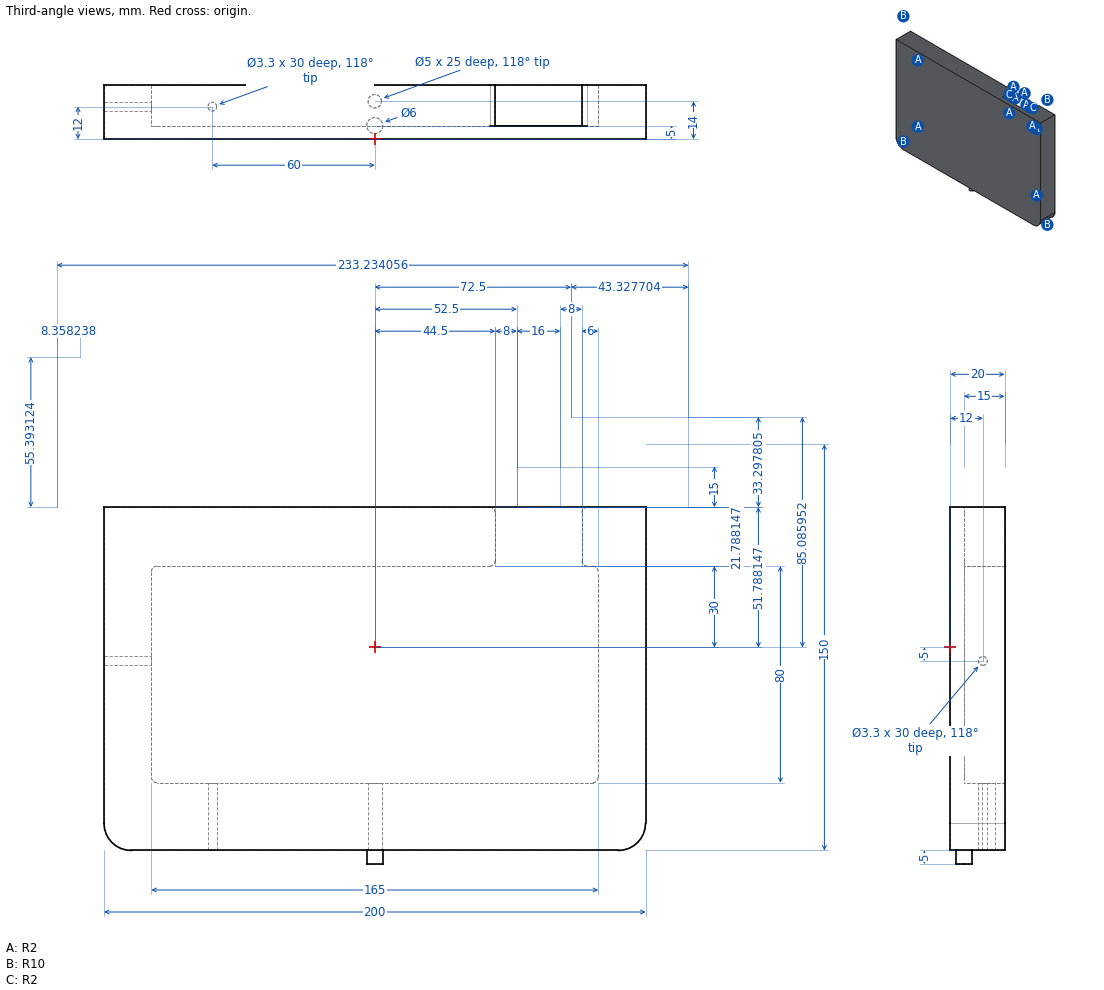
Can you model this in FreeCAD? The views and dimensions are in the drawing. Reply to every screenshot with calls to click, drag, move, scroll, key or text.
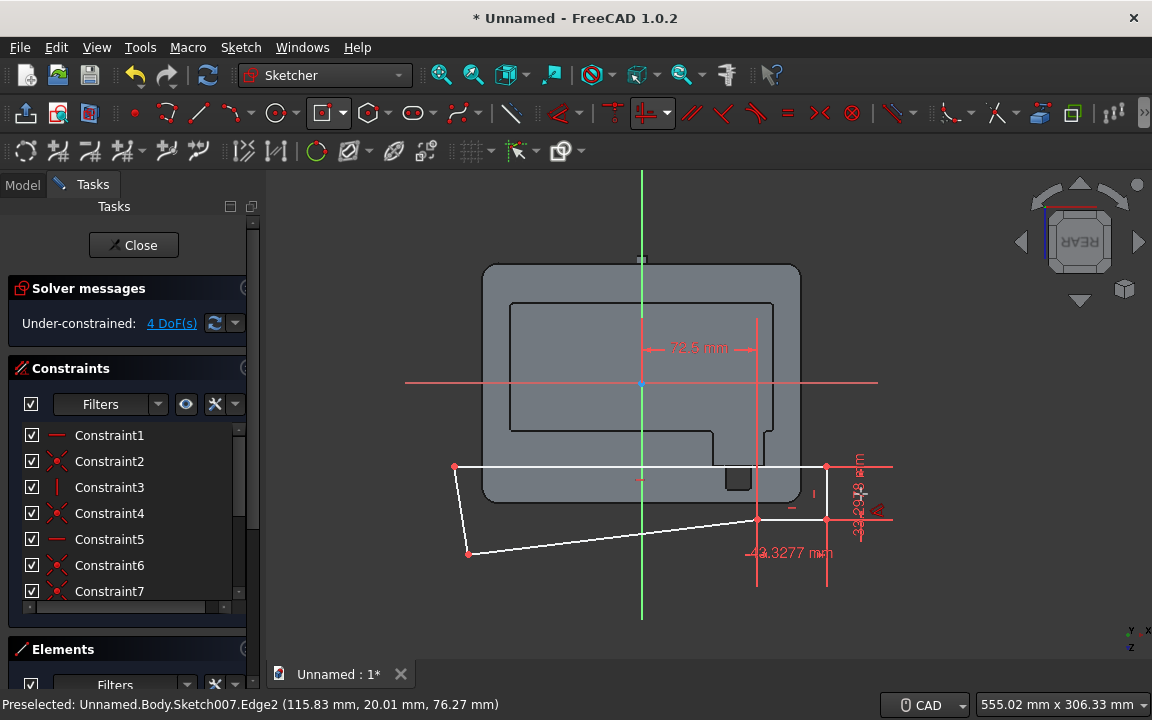
scroll(458, 493, up, 6)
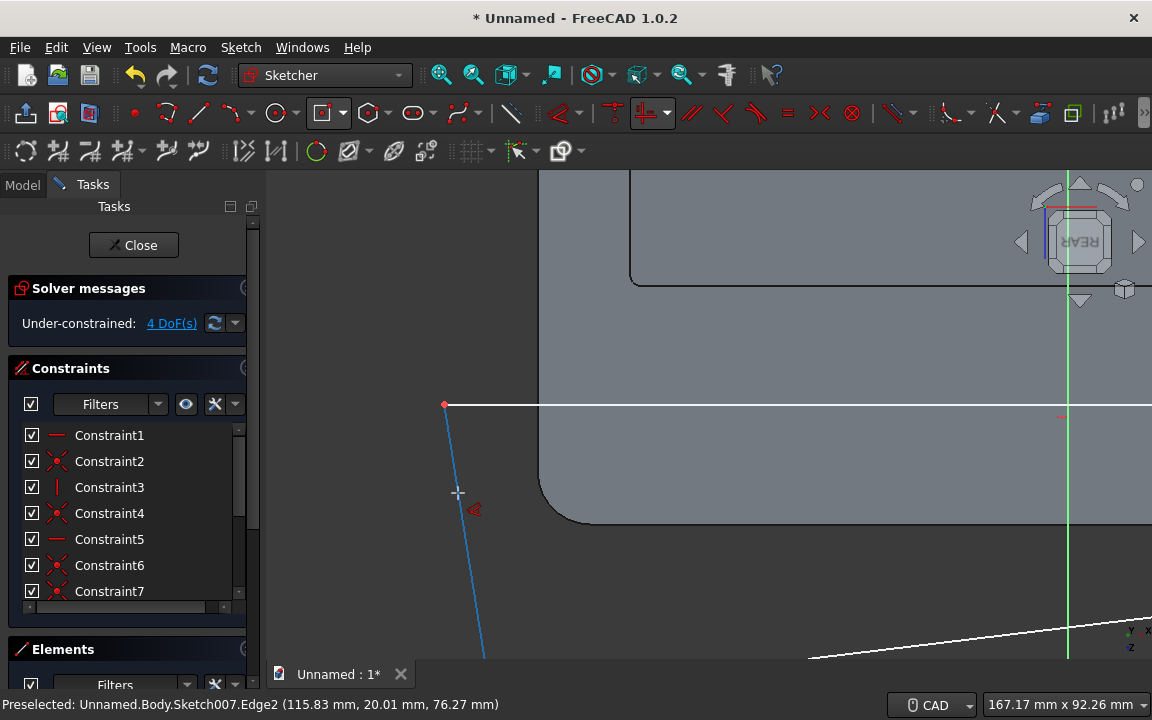
click(458, 492)
click(467, 371)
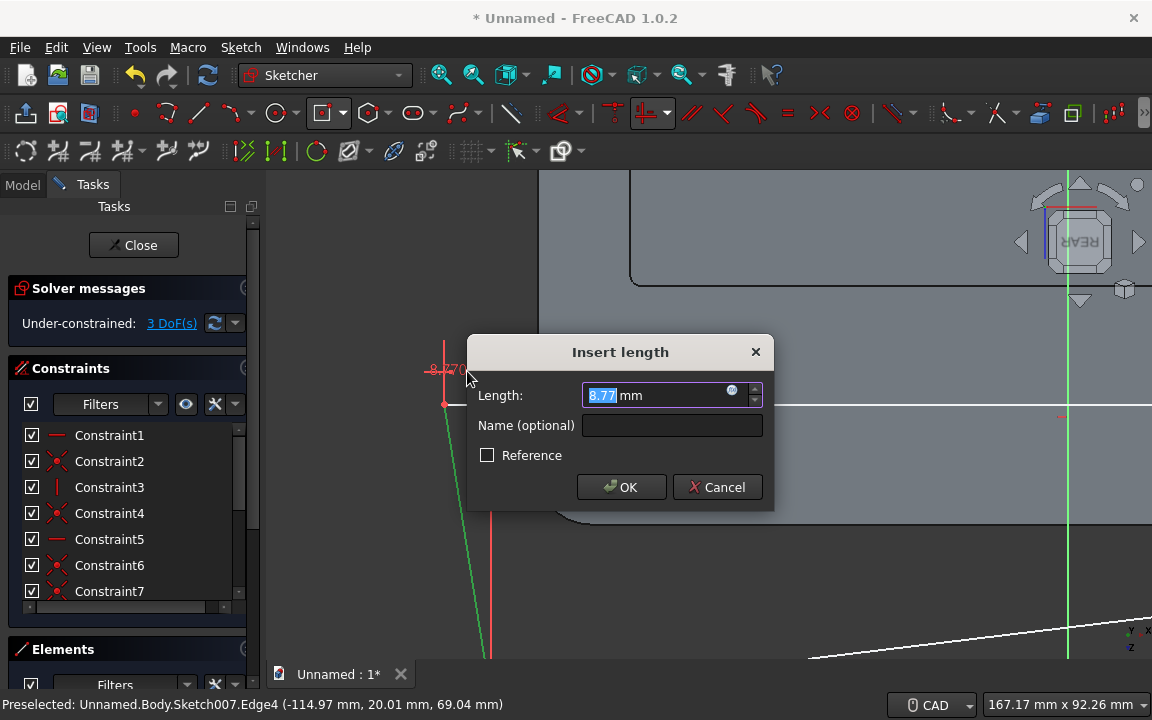
text(8.358238)
key(Return)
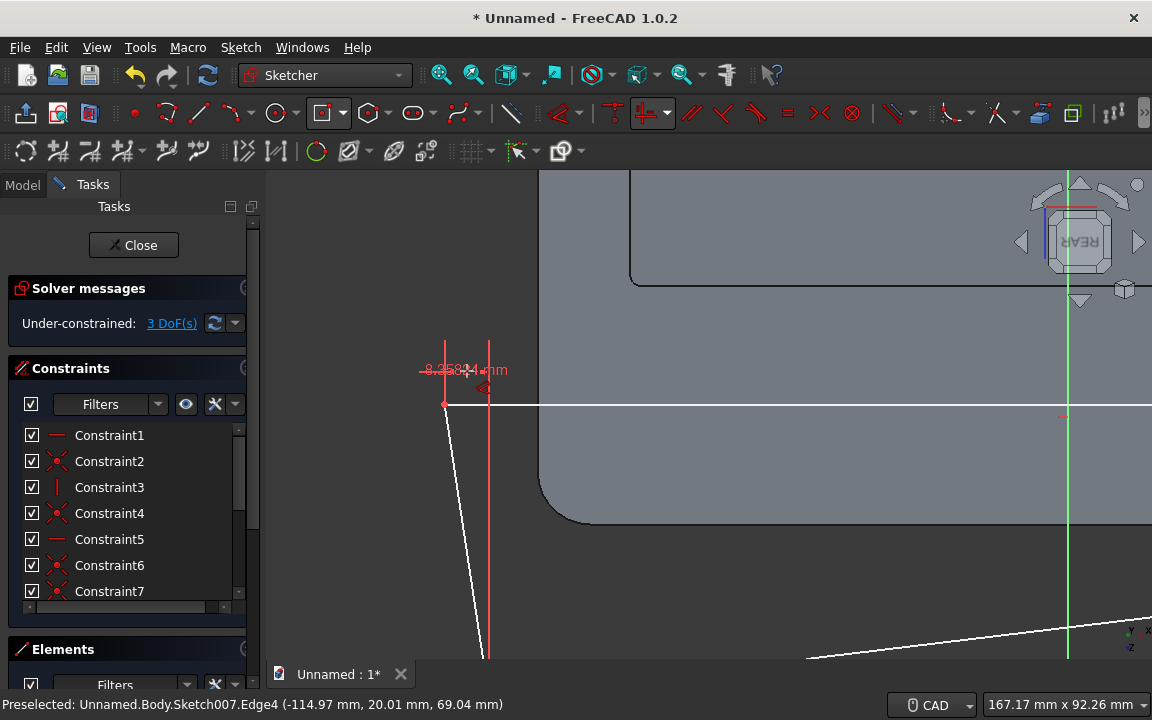
click(816, 405)
click(716, 371)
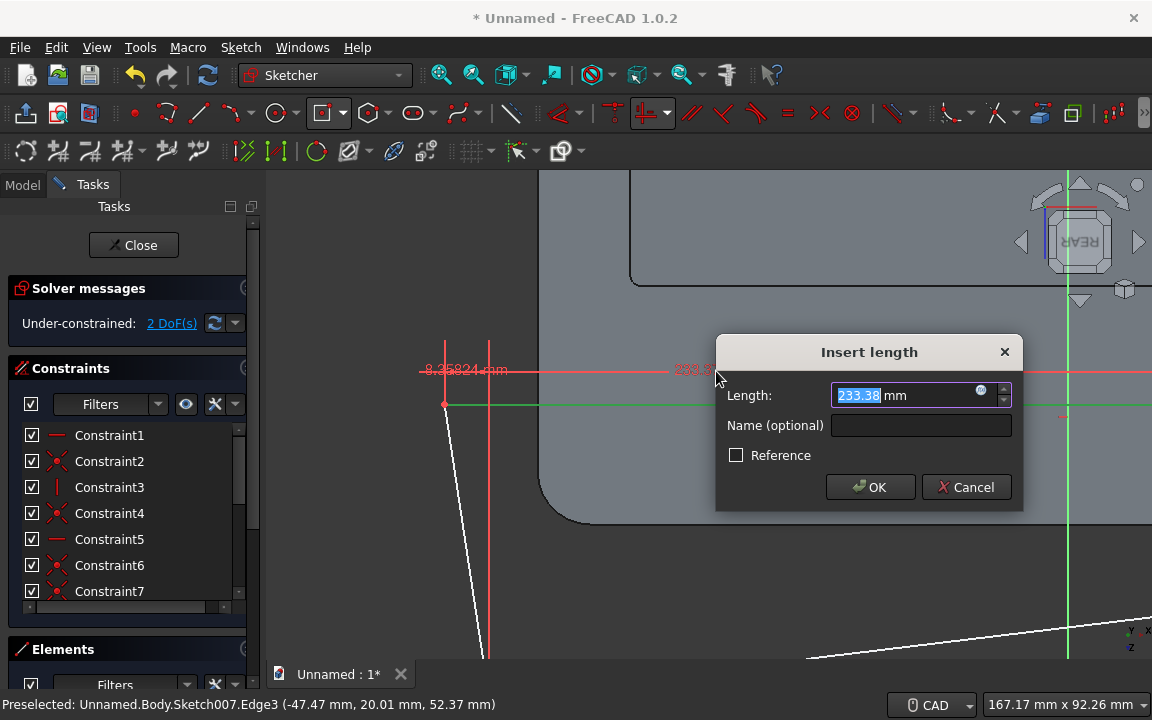
text(233.234056)
key(Return)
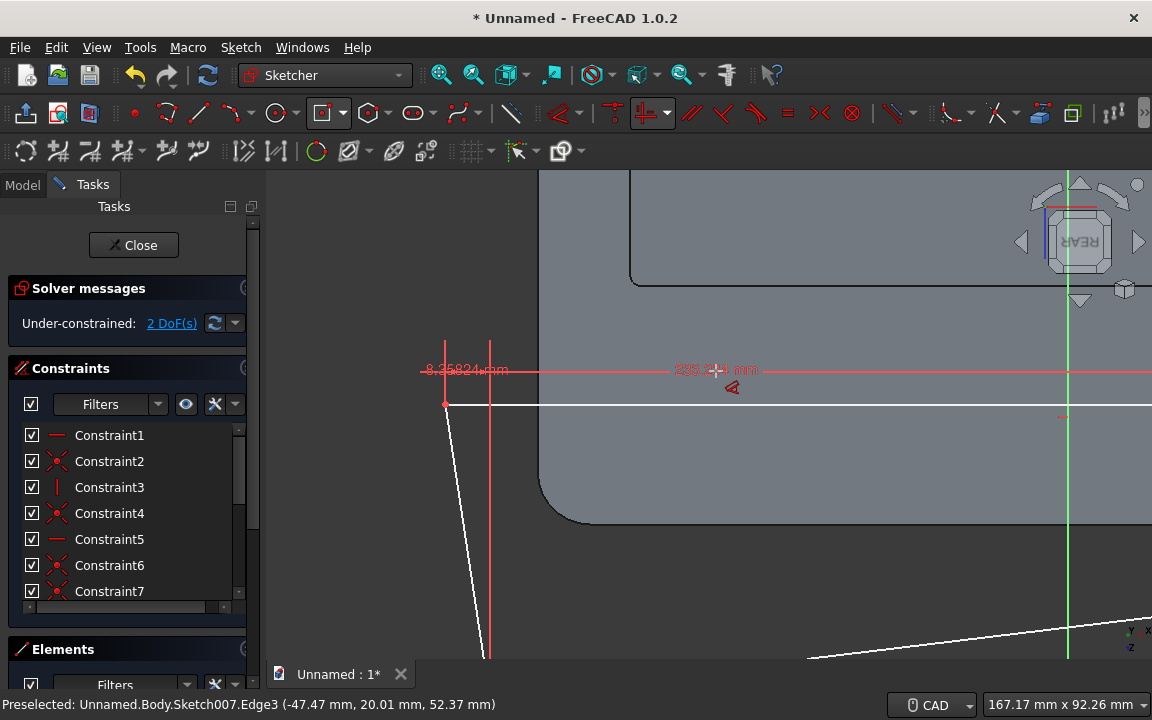
scroll(394, 416, down, 5)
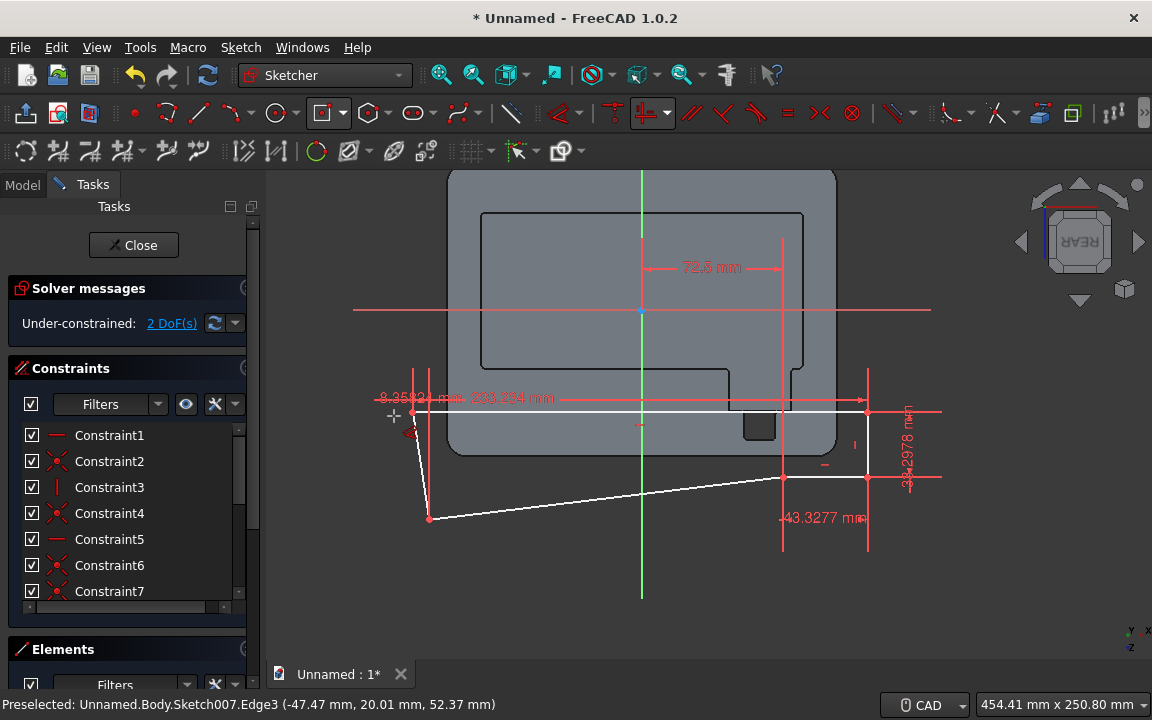
click(783, 477)
click(817, 394)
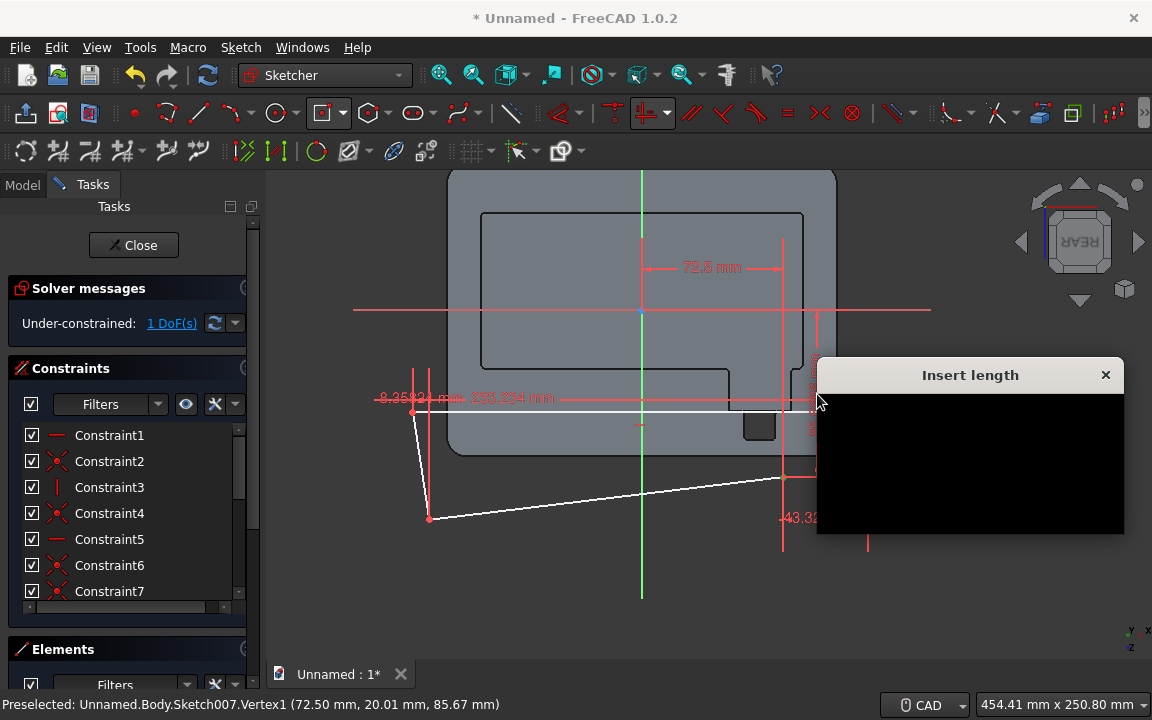
text(85.085952)
key(Return)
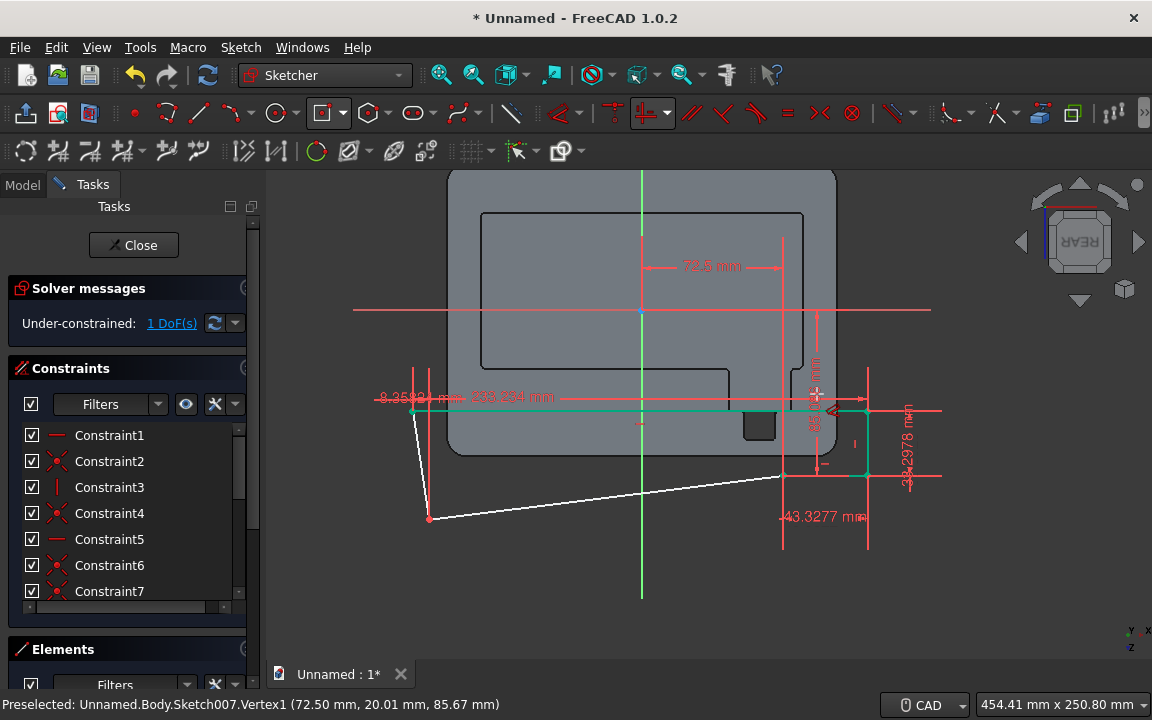
click(418, 444)
click(379, 465)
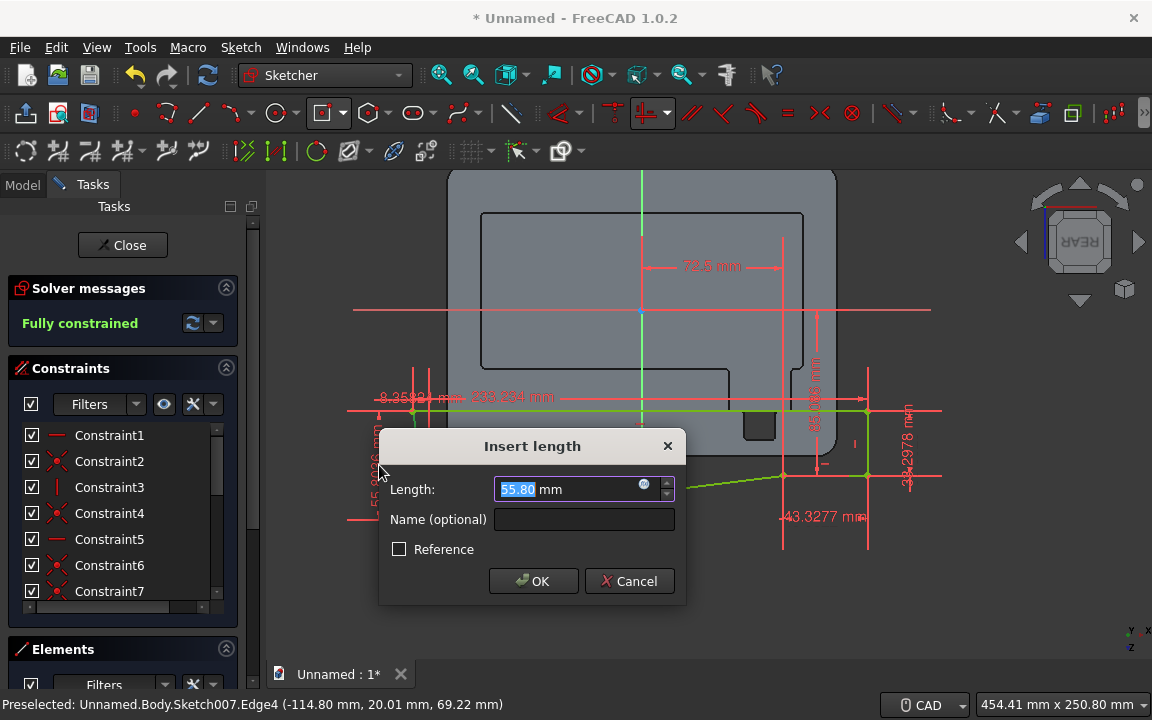
text(55.393124)
key(Return)
key(Escape)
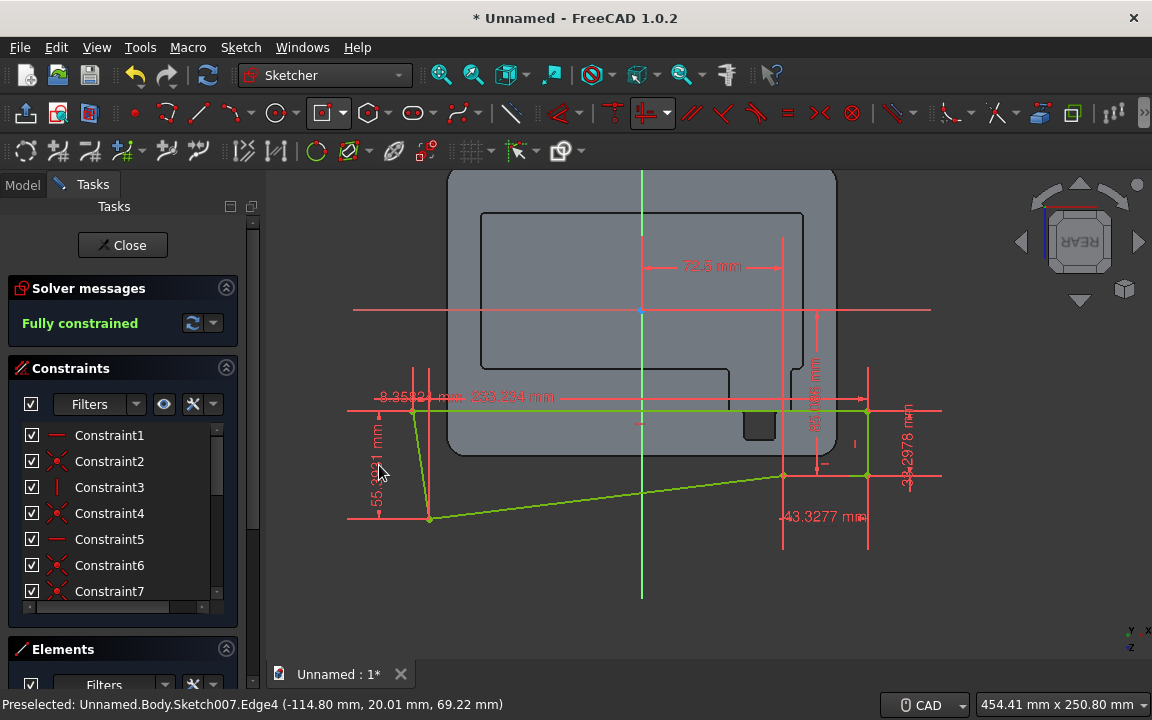
click(123, 245)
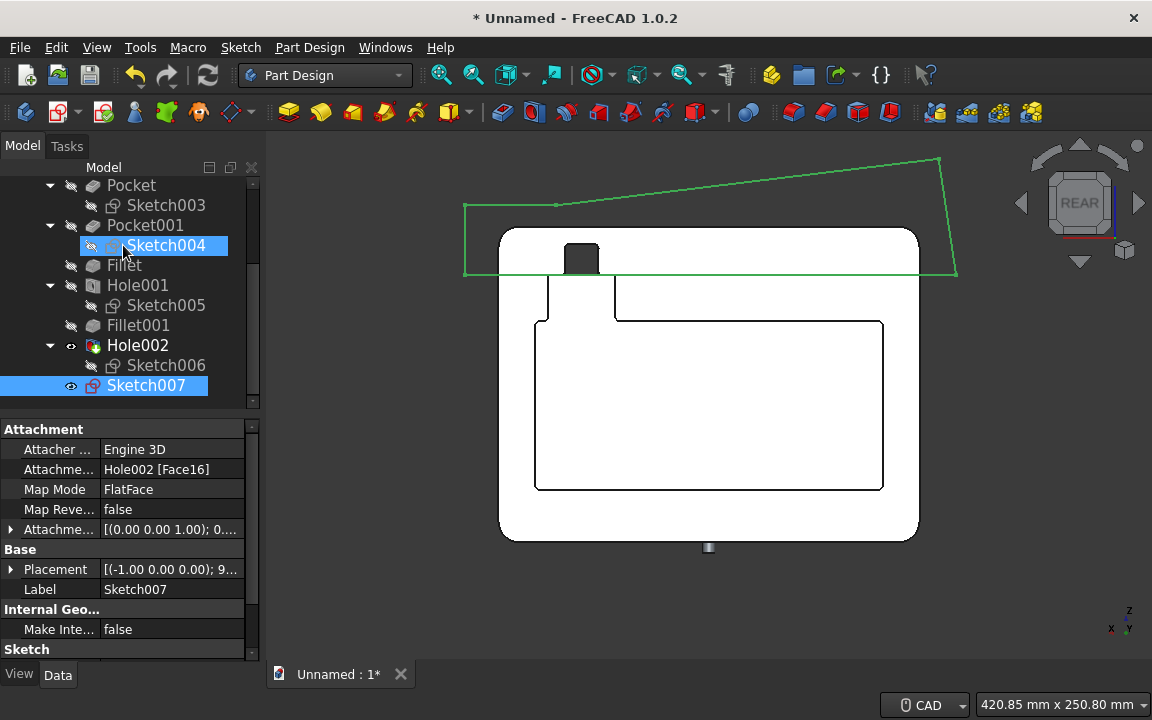
click(504, 112)